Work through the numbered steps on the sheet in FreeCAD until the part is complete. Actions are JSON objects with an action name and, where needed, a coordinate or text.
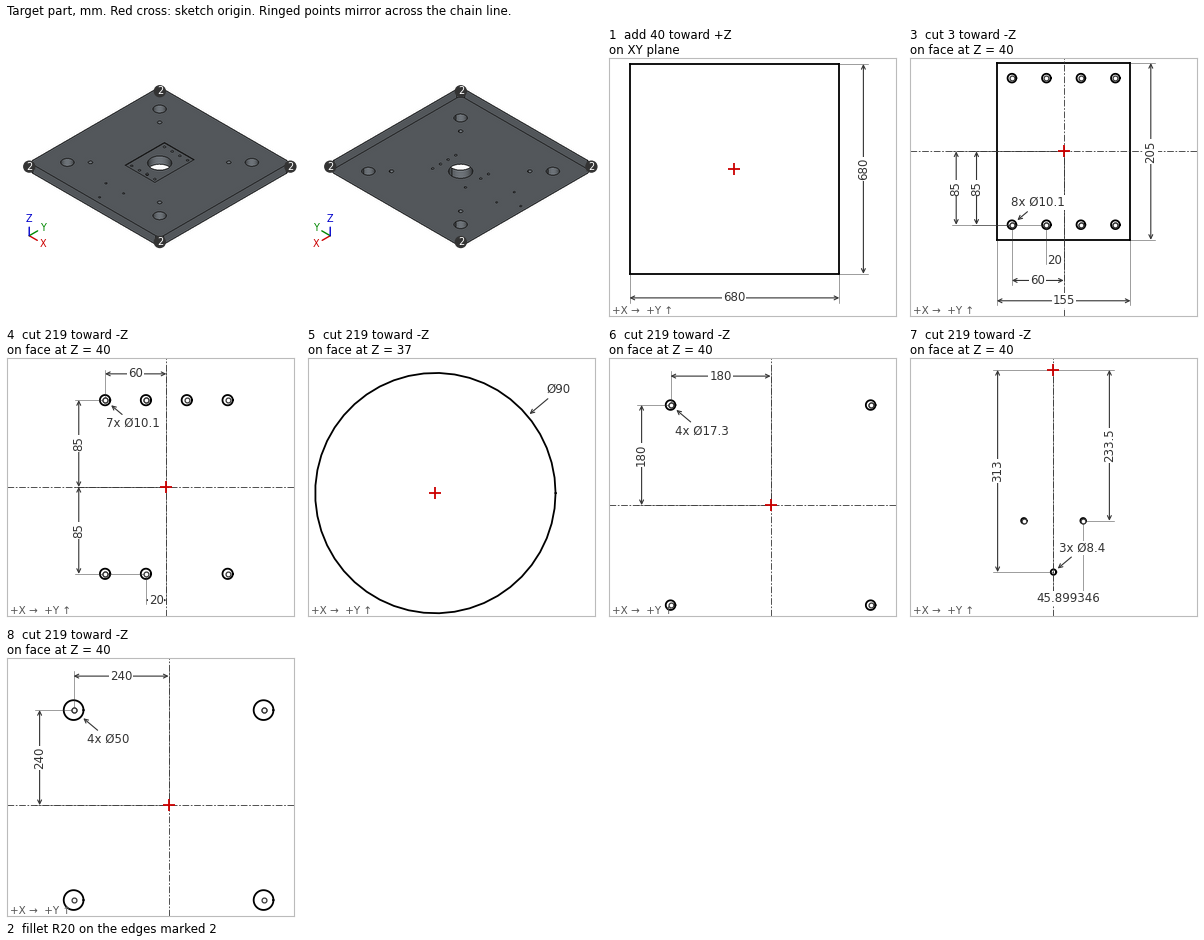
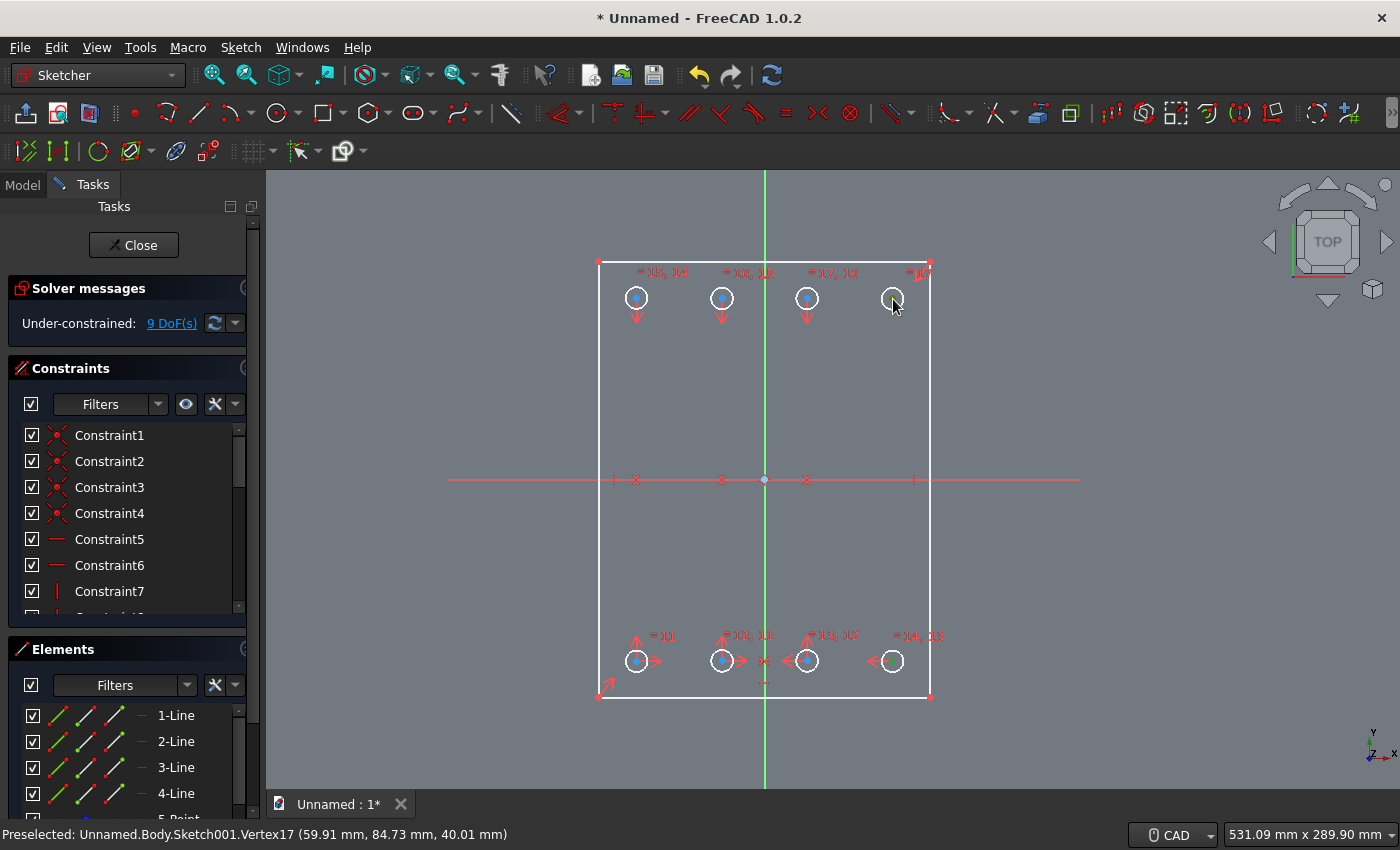
{"action": "left_click", "coordinate": [496, 480]}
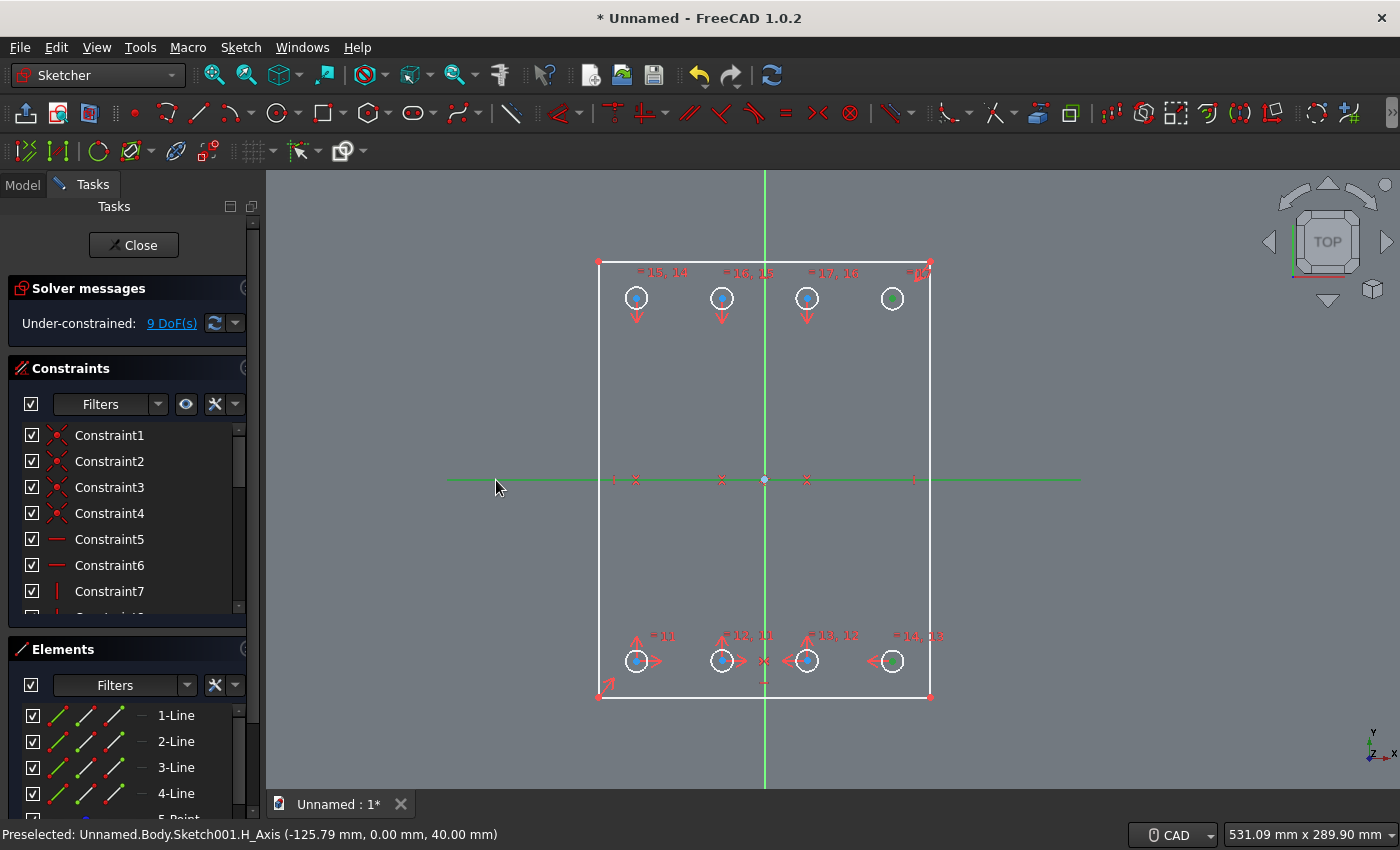
{"action": "left_click", "coordinate": [818, 114]}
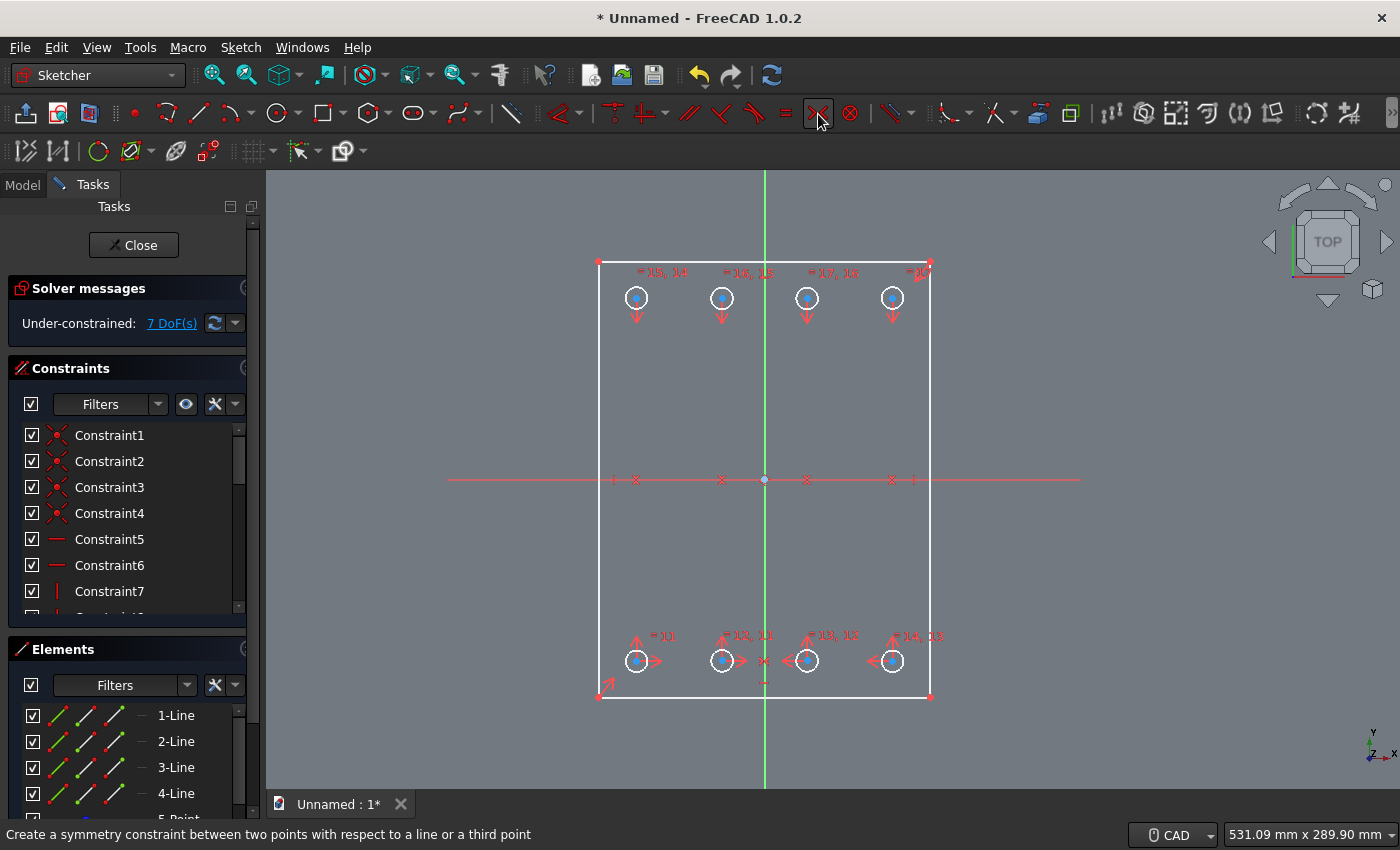
{"action": "left_click", "coordinate": [558, 114]}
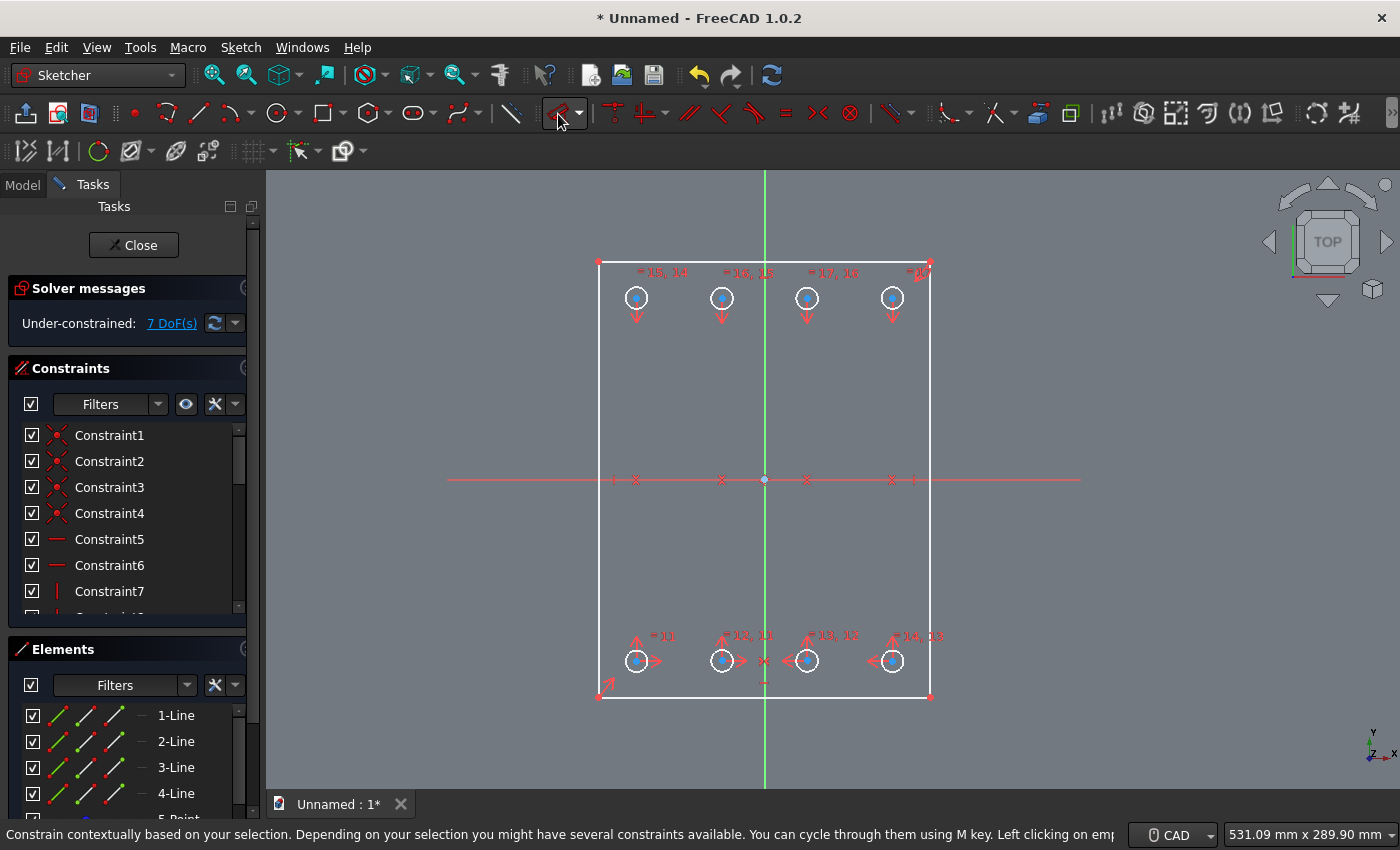
{"action": "scroll", "coordinate": [644, 654], "scroll_direction": "up", "scroll_amount": 4}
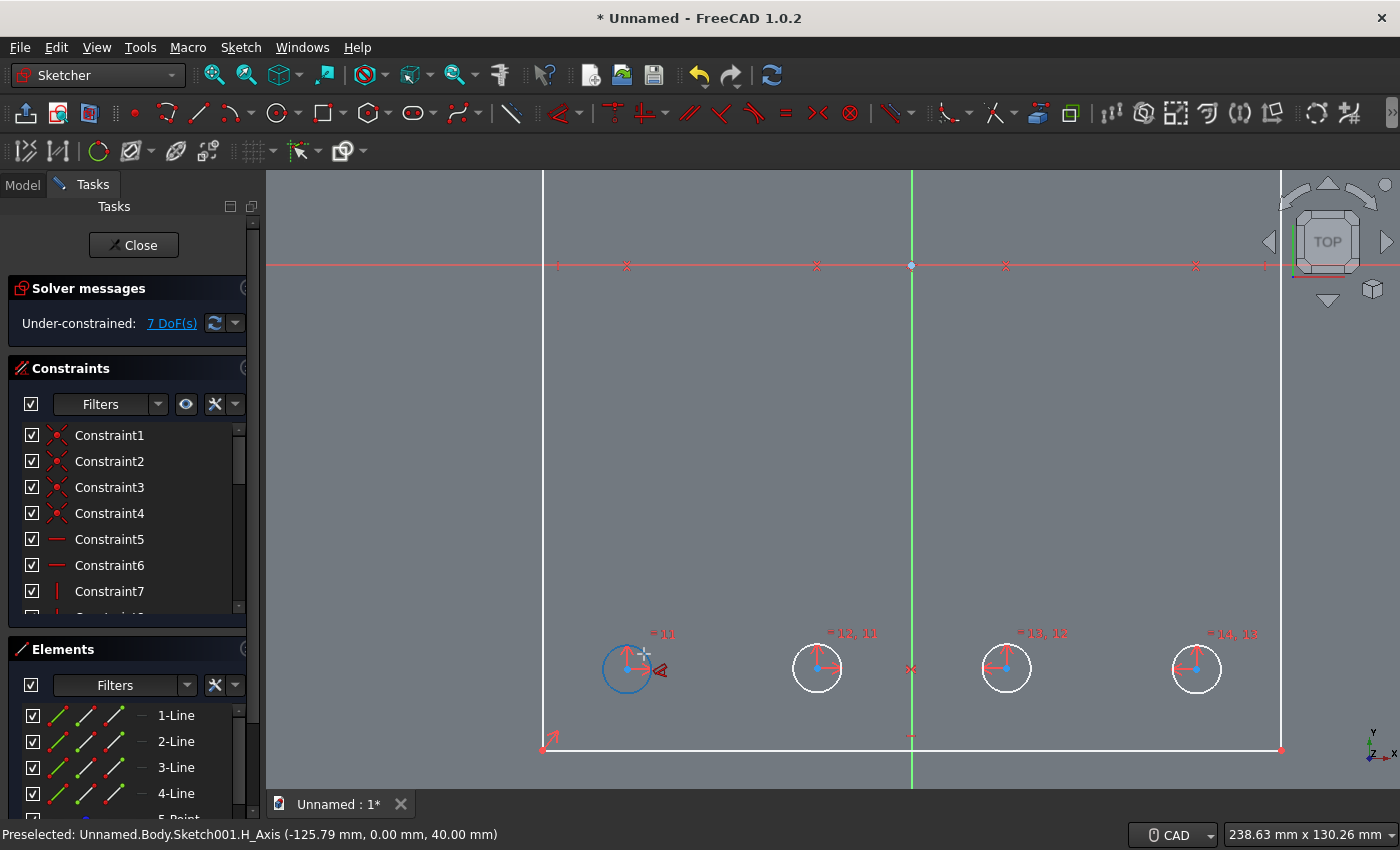
{"action": "left_click", "coordinate": [644, 652]}
{"action": "left_click", "coordinate": [666, 629]}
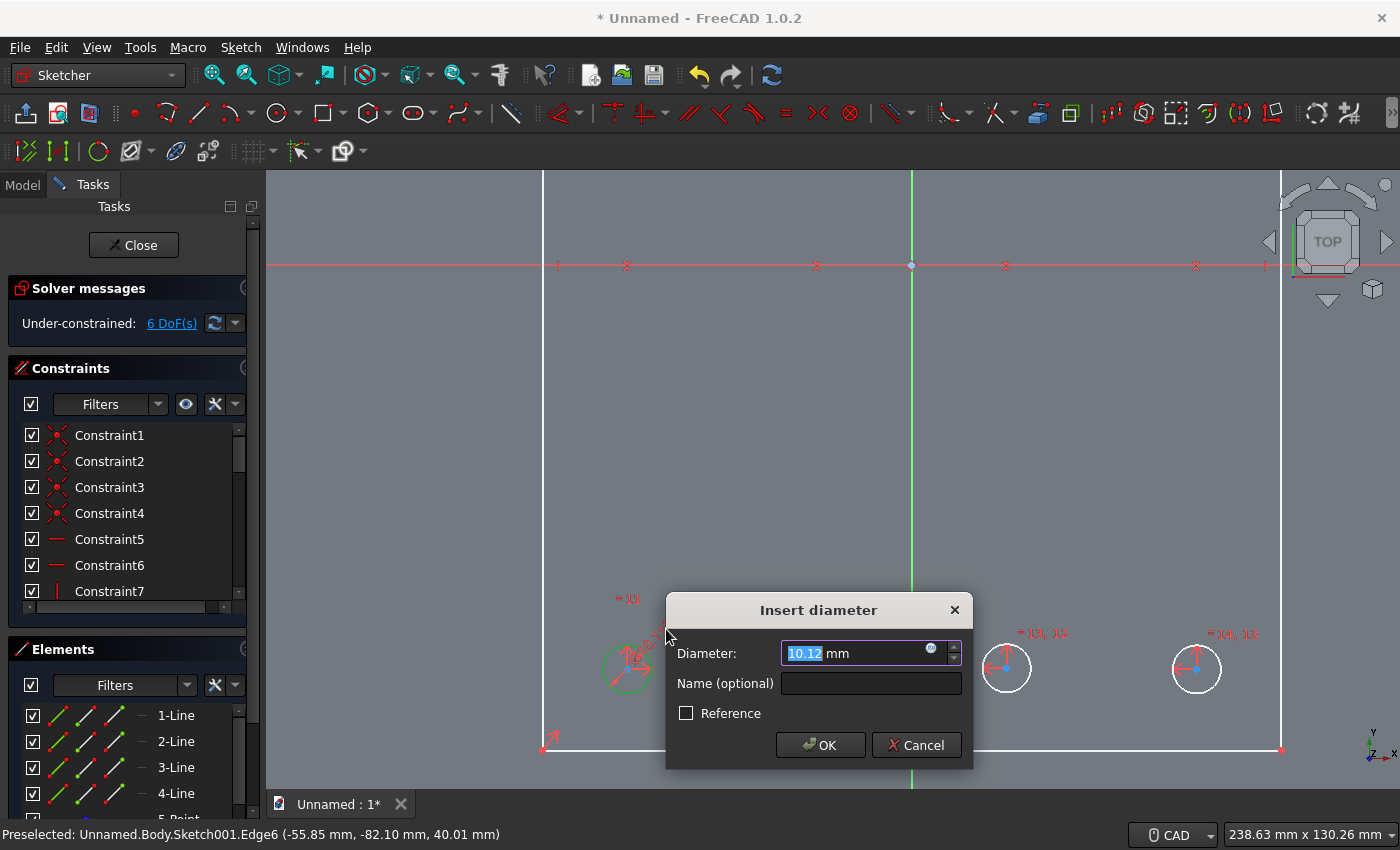
{"action": "type", "text": "10.1"}
{"action": "key", "text": "Return"}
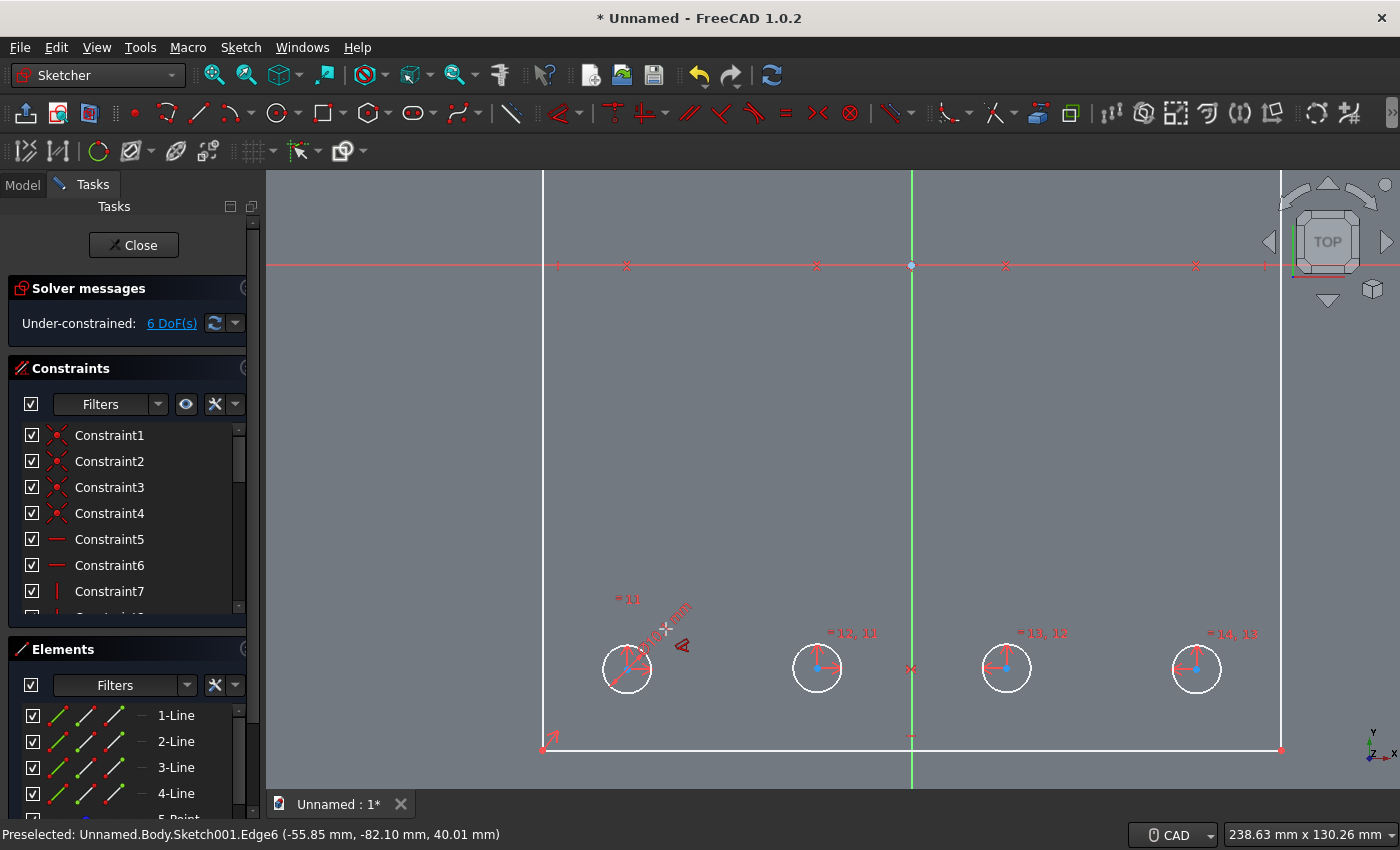
{"action": "left_click", "coordinate": [627, 669]}
{"action": "left_click", "coordinate": [770, 703]}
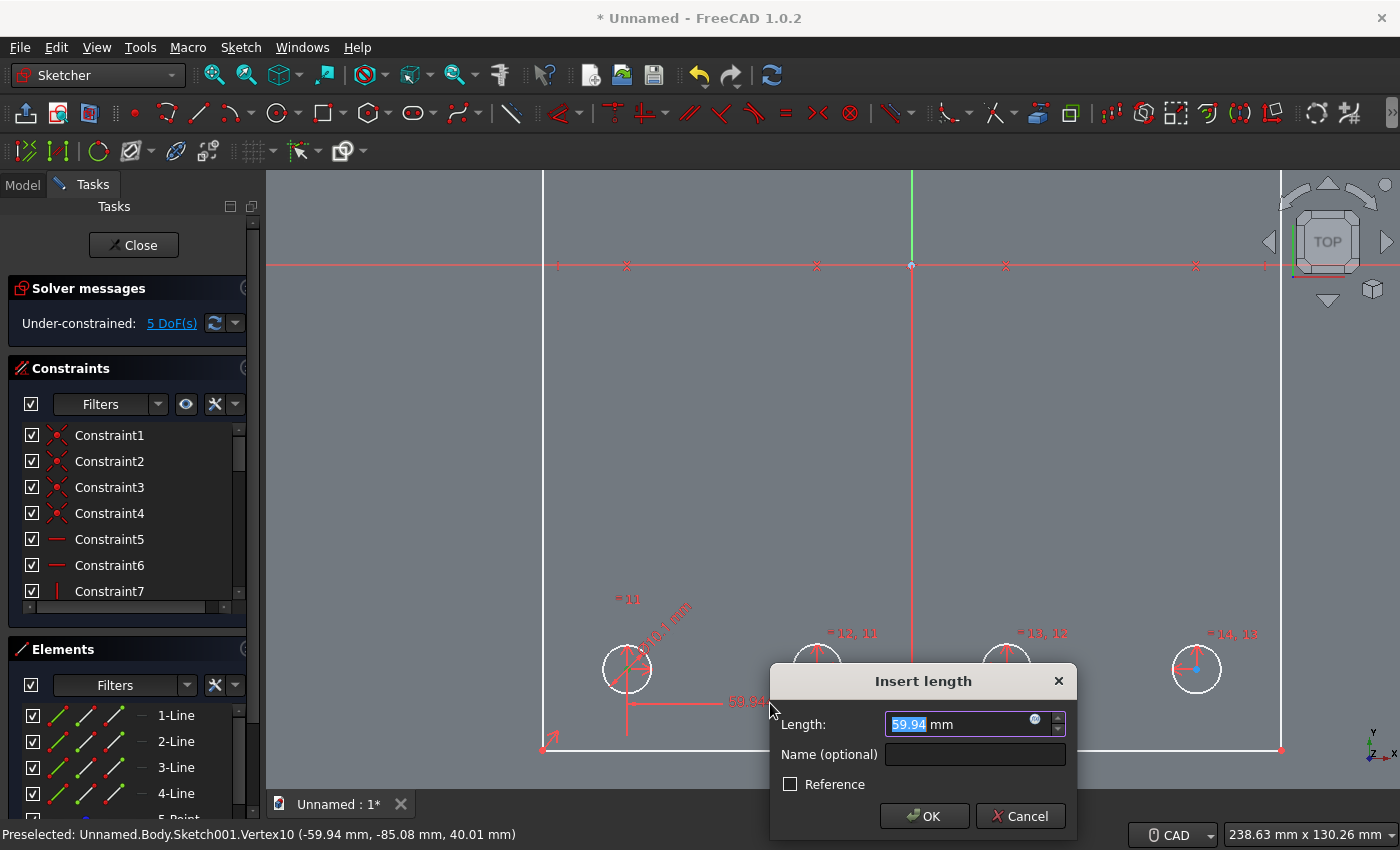
{"action": "type", "text": "60"}
{"action": "key", "text": "Return"}